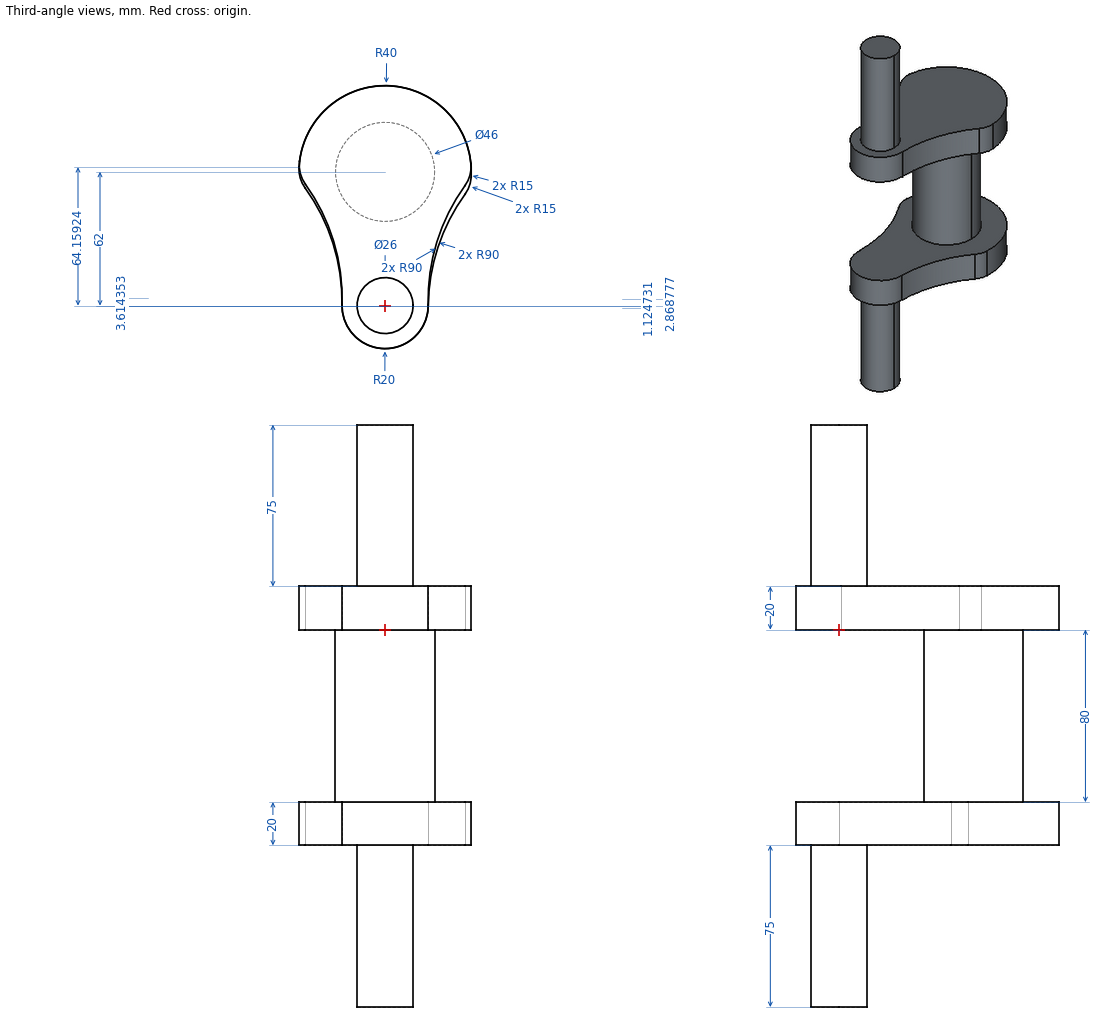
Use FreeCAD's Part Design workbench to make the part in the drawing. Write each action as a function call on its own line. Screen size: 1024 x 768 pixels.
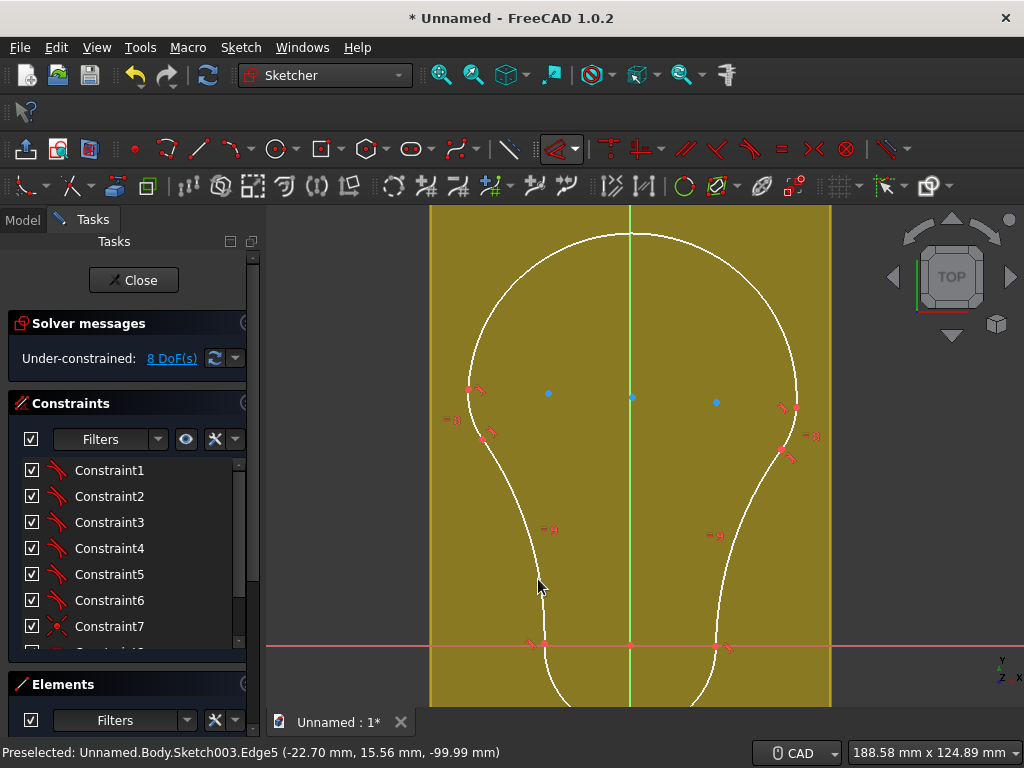
click(632, 398)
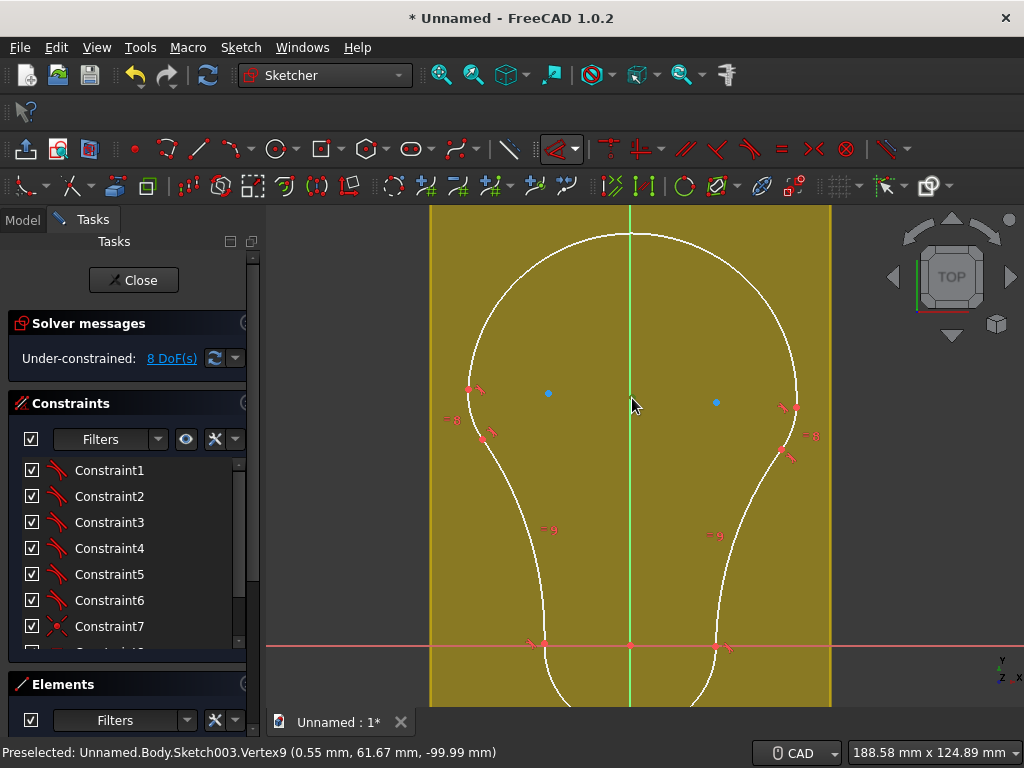
click(630, 615)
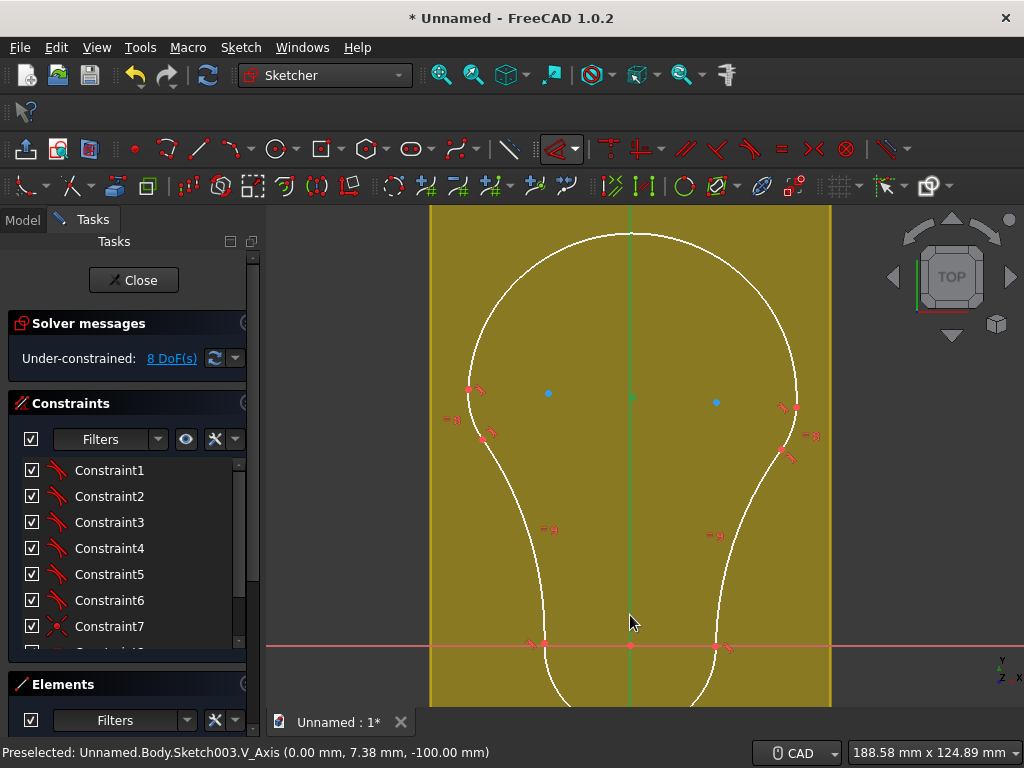
click(610, 150)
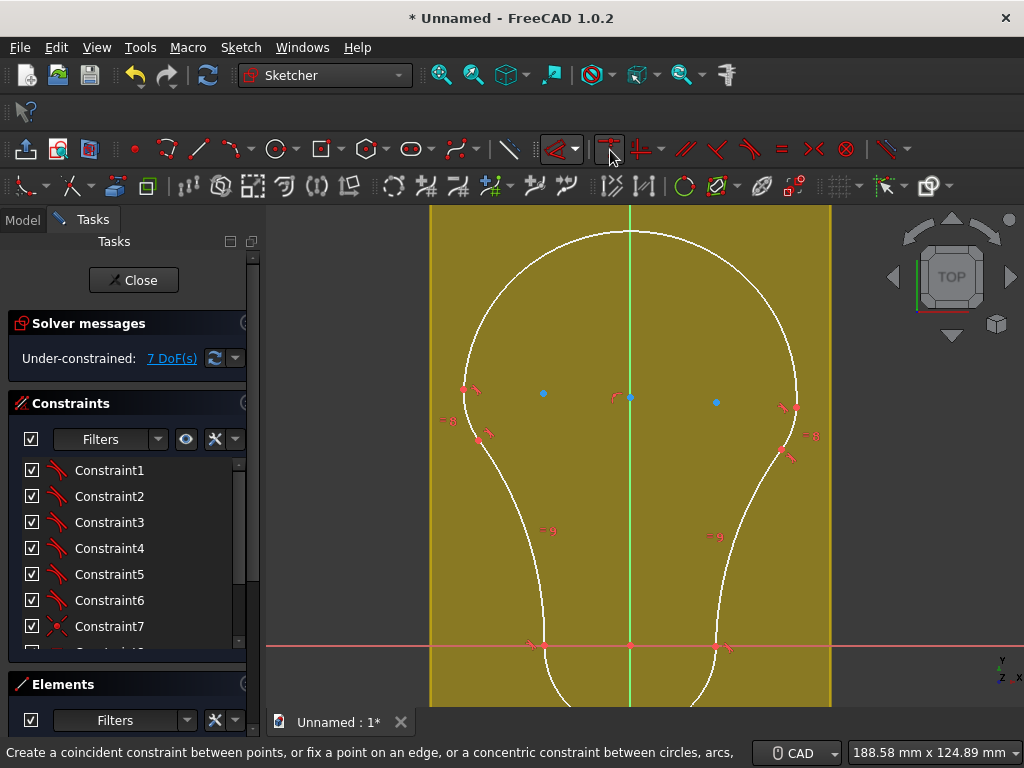
click(749, 504)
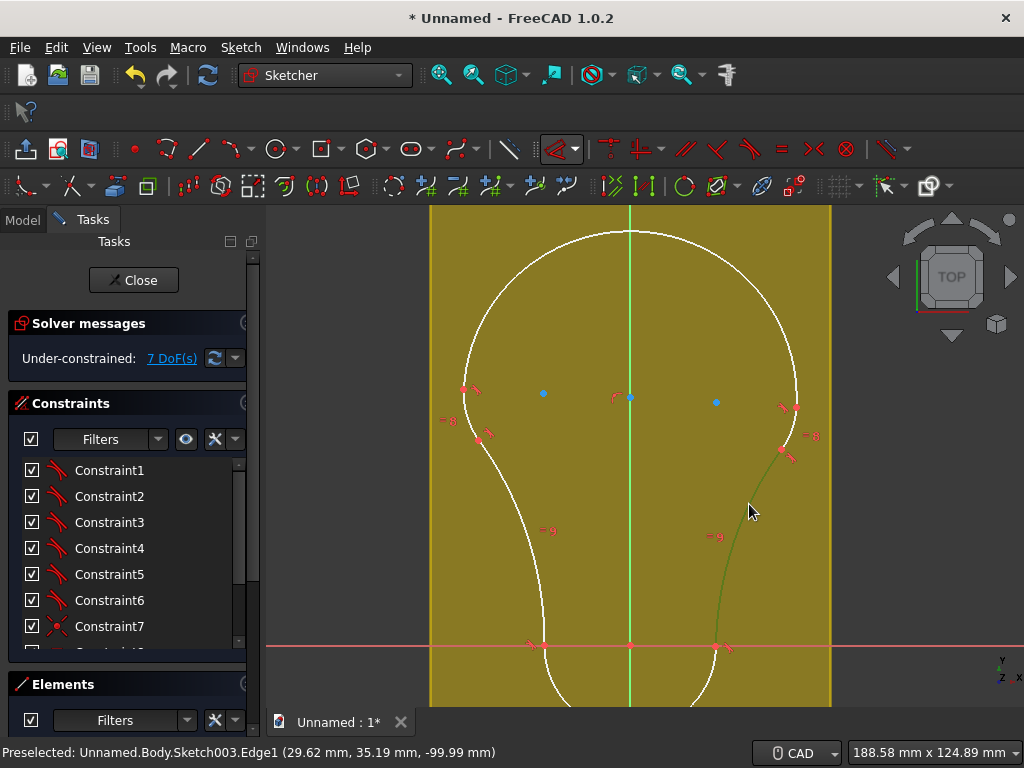
click(578, 150)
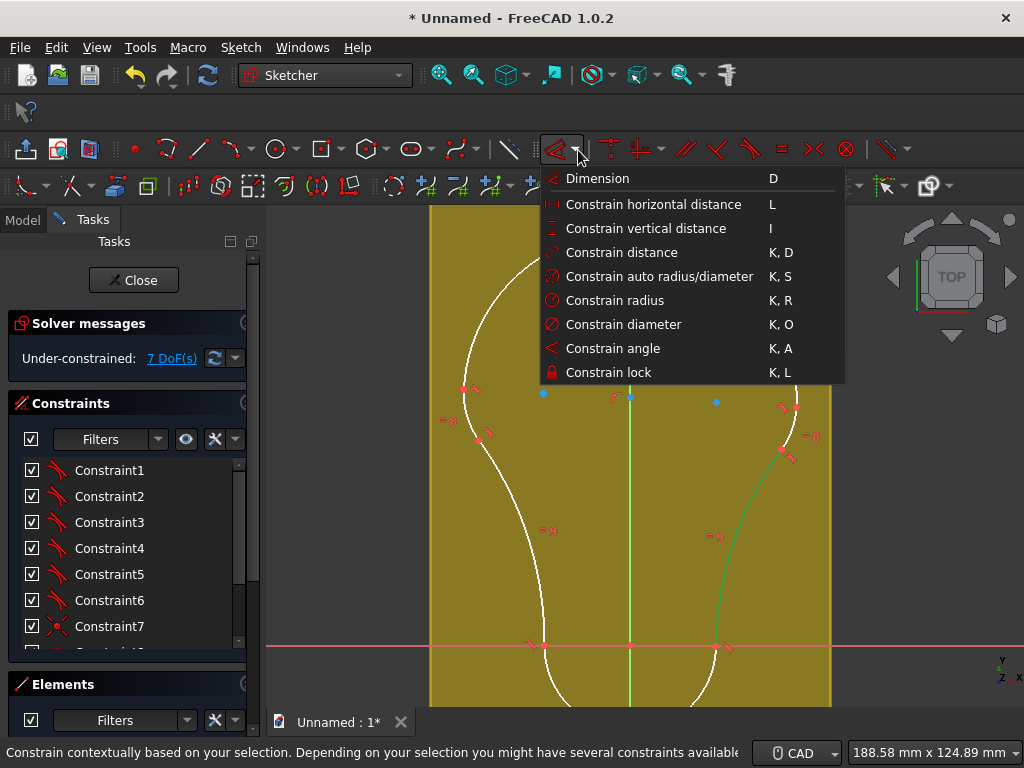
click(693, 300)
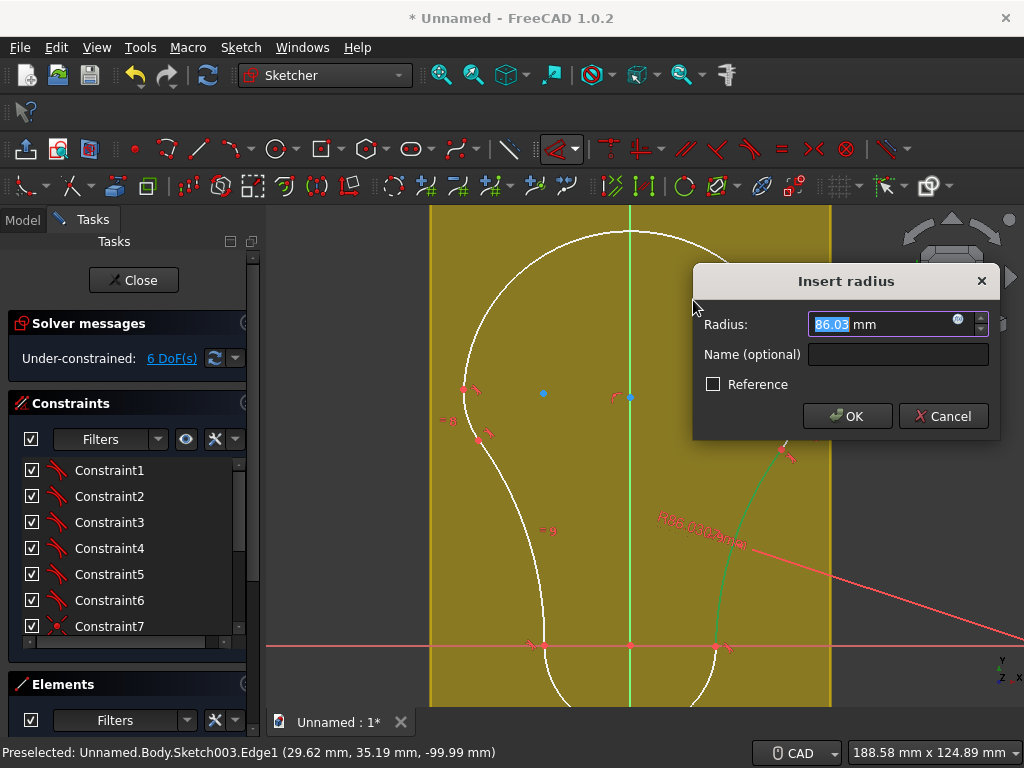
text(90)
key(Return)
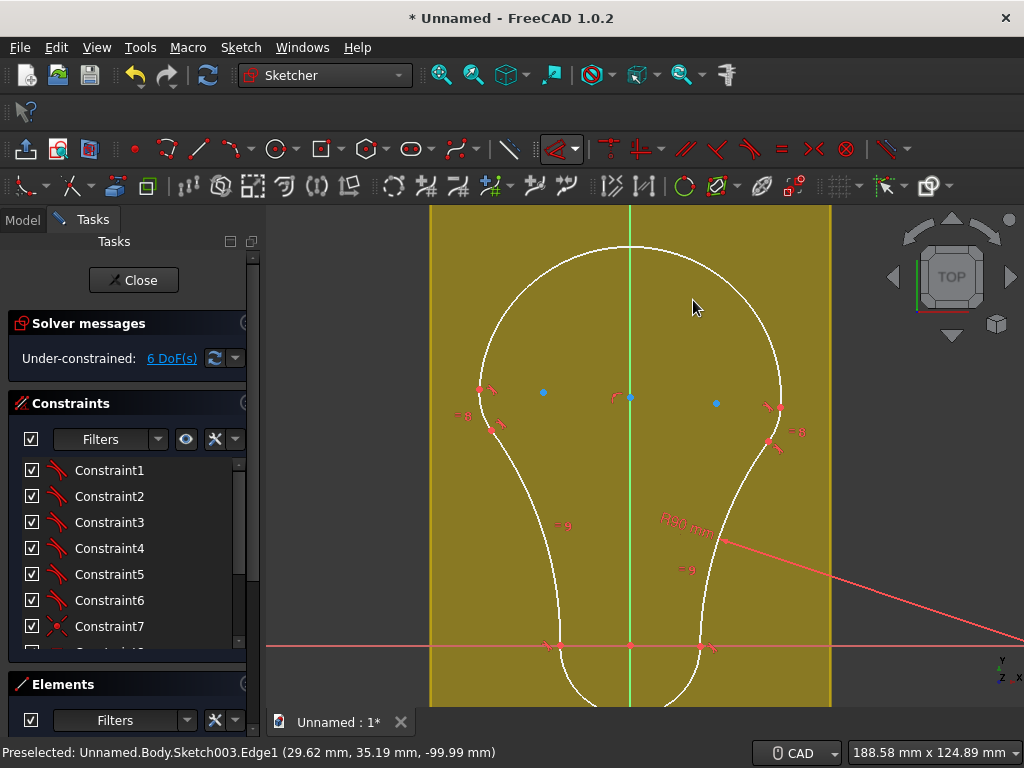
scroll(774, 432, up, 2)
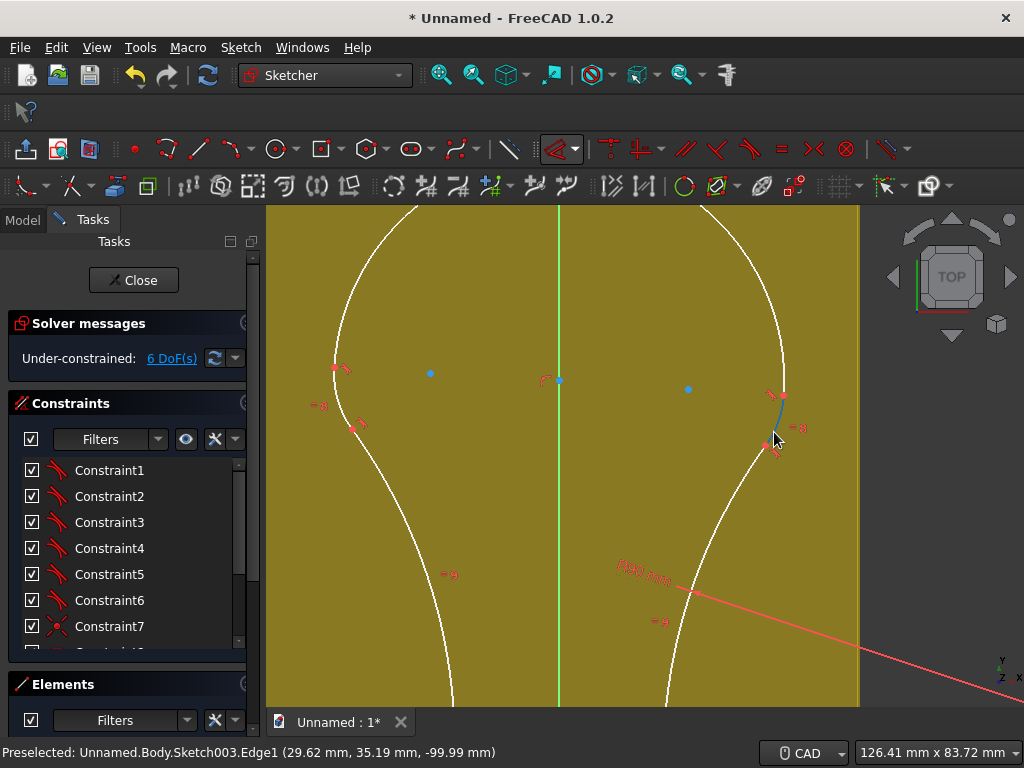
click(774, 432)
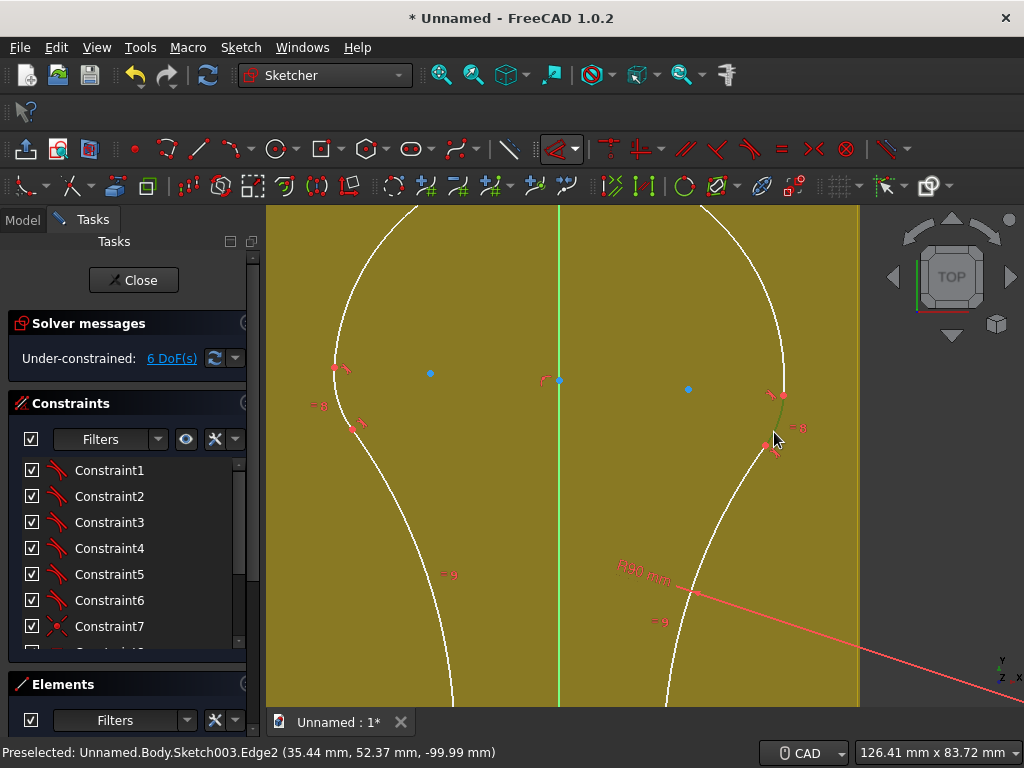
key(k)
key(r)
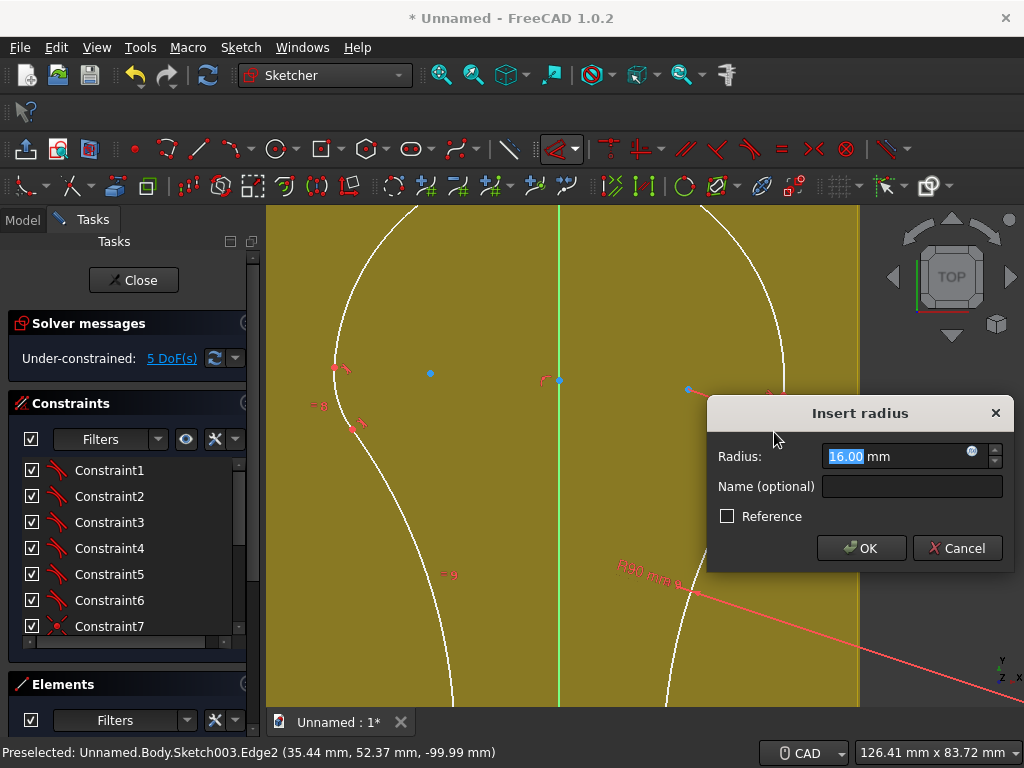
text(15)
key(Return)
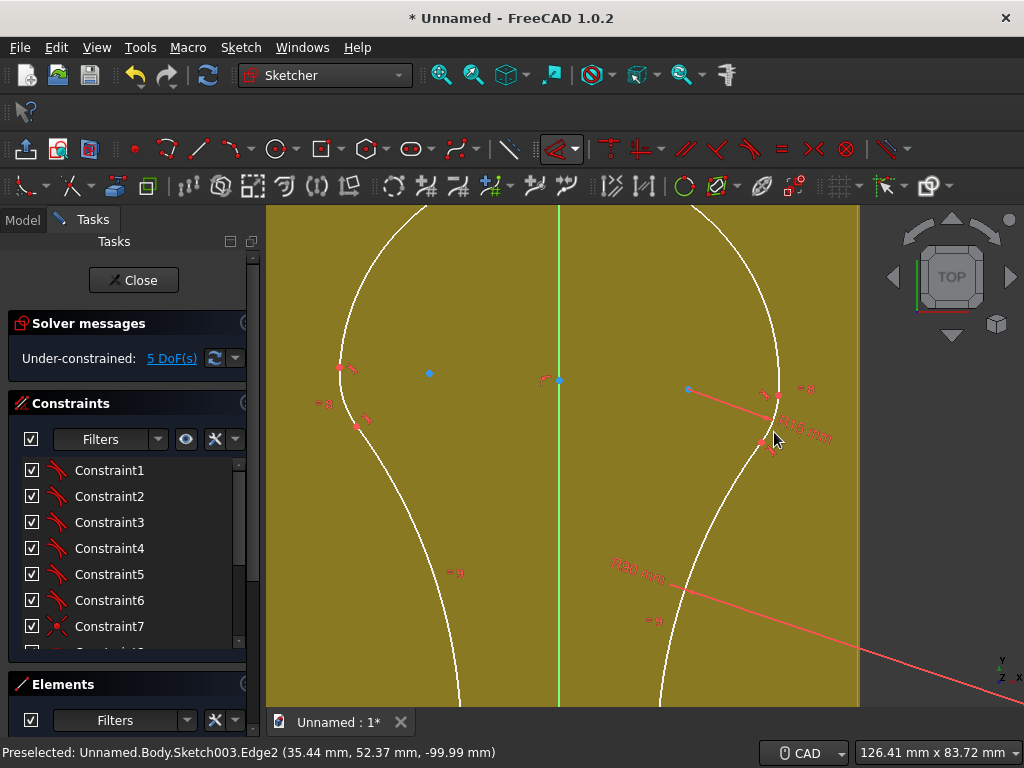
click(745, 264)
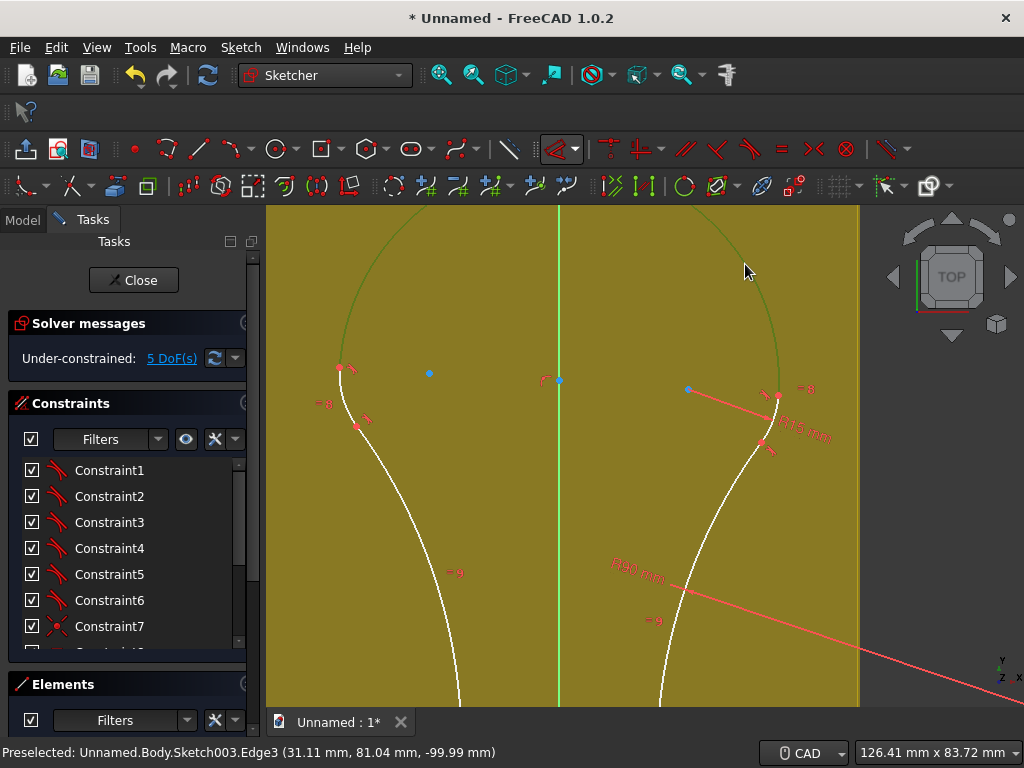
click(578, 150)